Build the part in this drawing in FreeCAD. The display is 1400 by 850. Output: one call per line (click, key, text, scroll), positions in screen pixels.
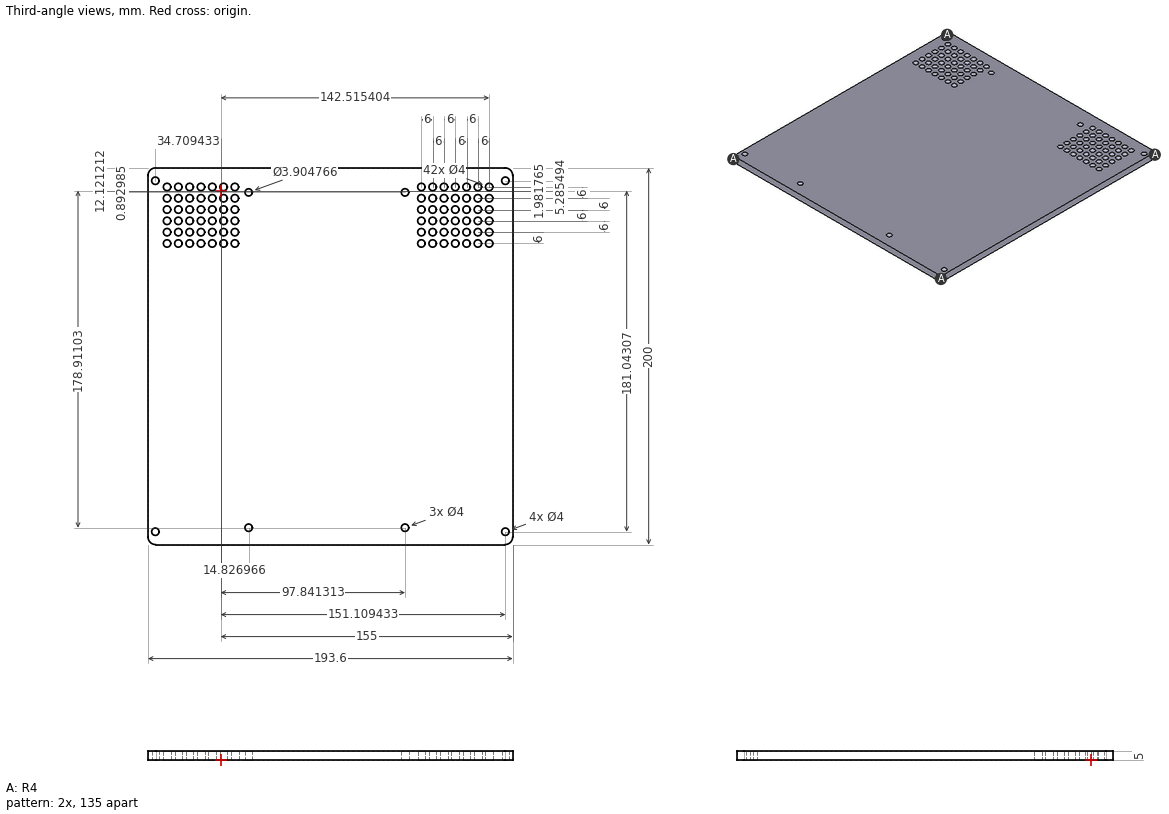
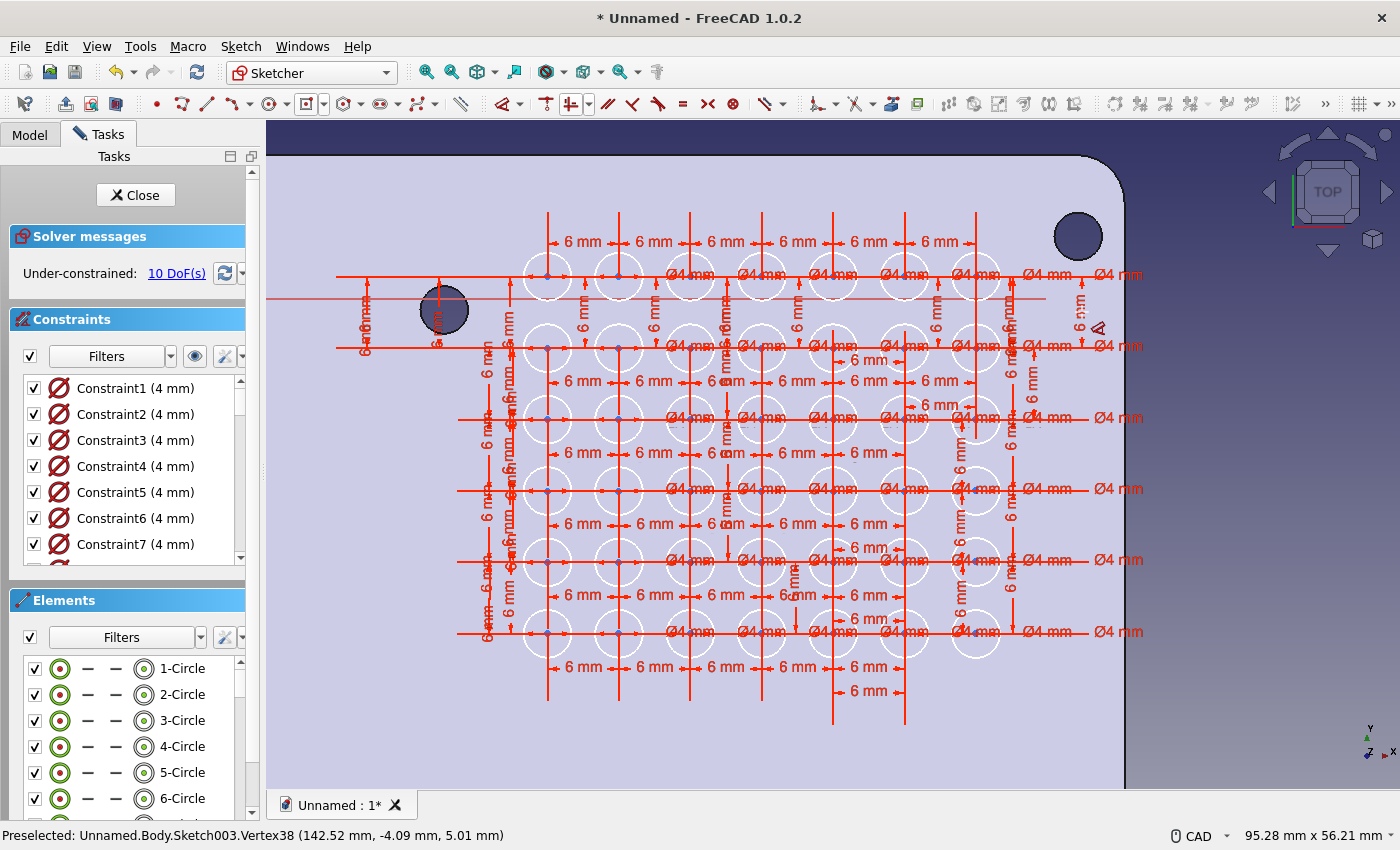
click(905, 420)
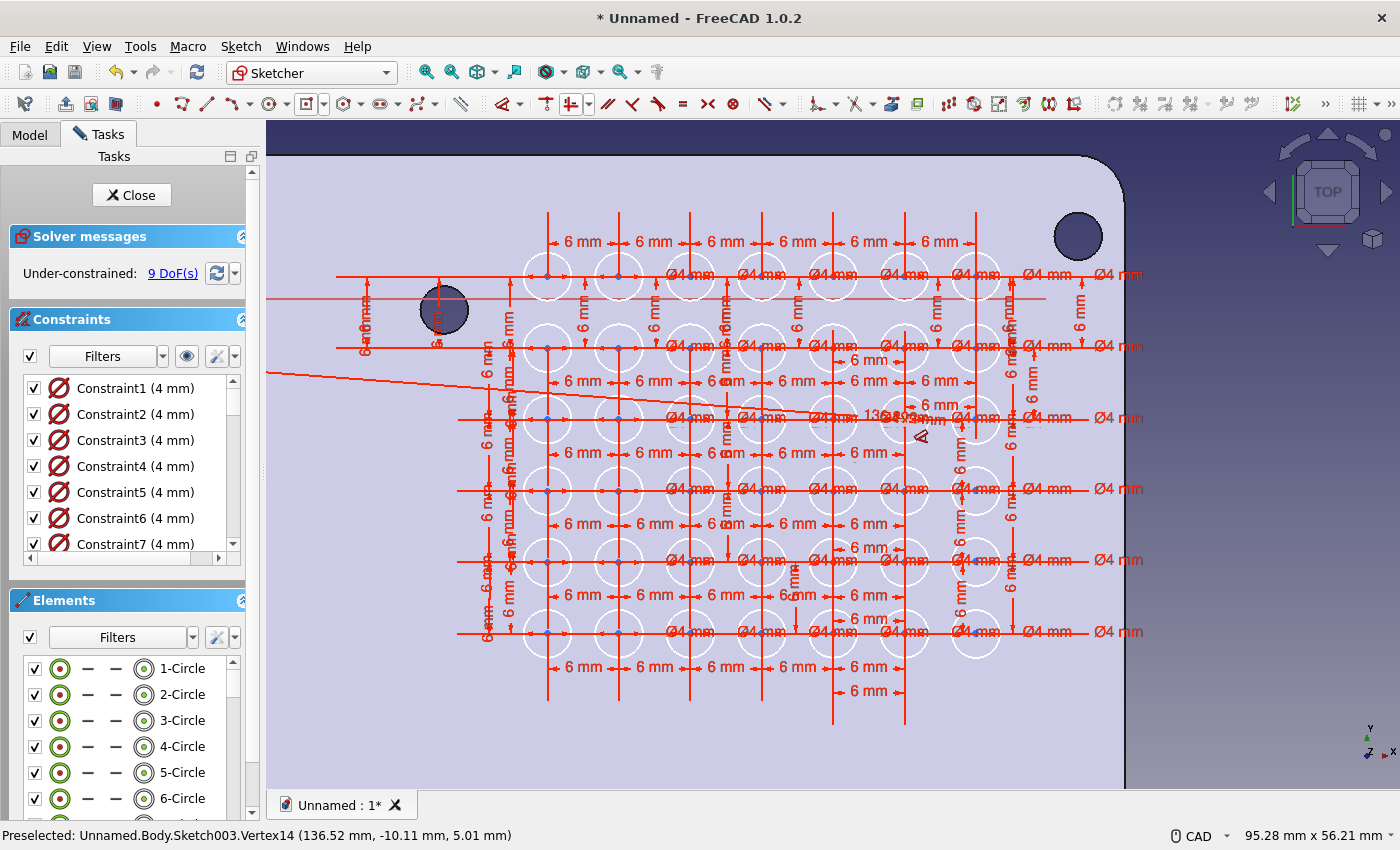
click(976, 420)
click(940, 362)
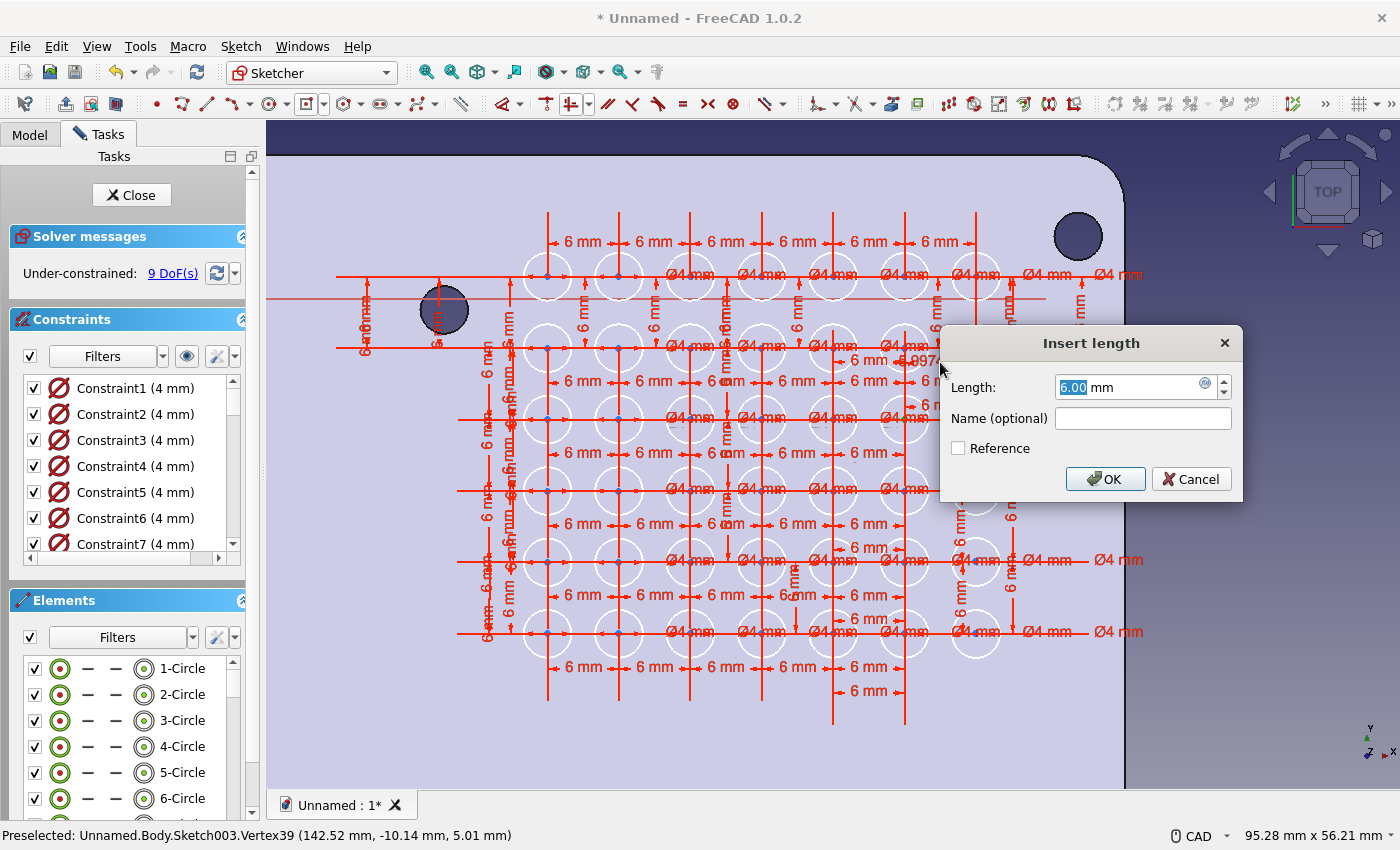
text(6)
key(Return)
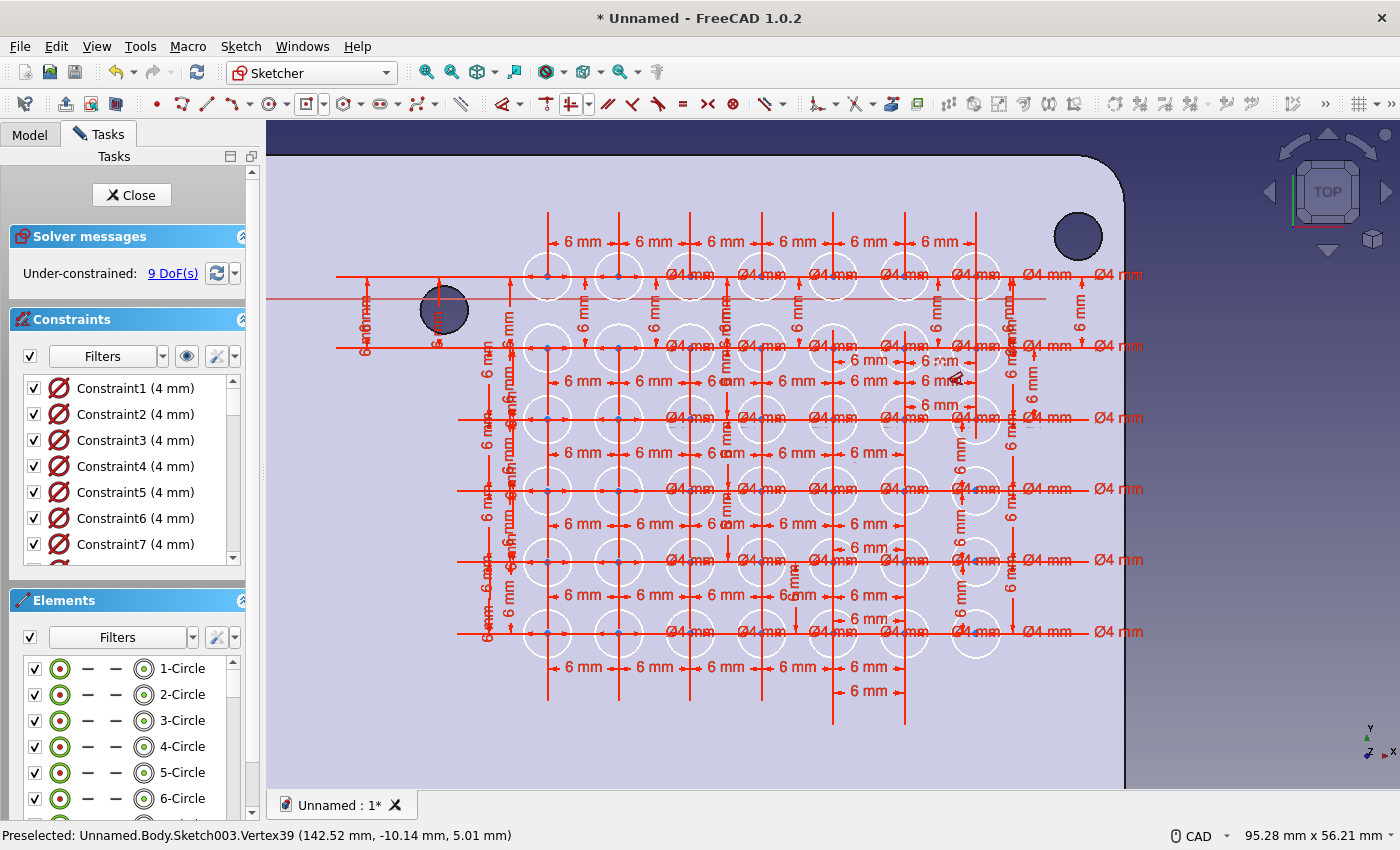
click(976, 348)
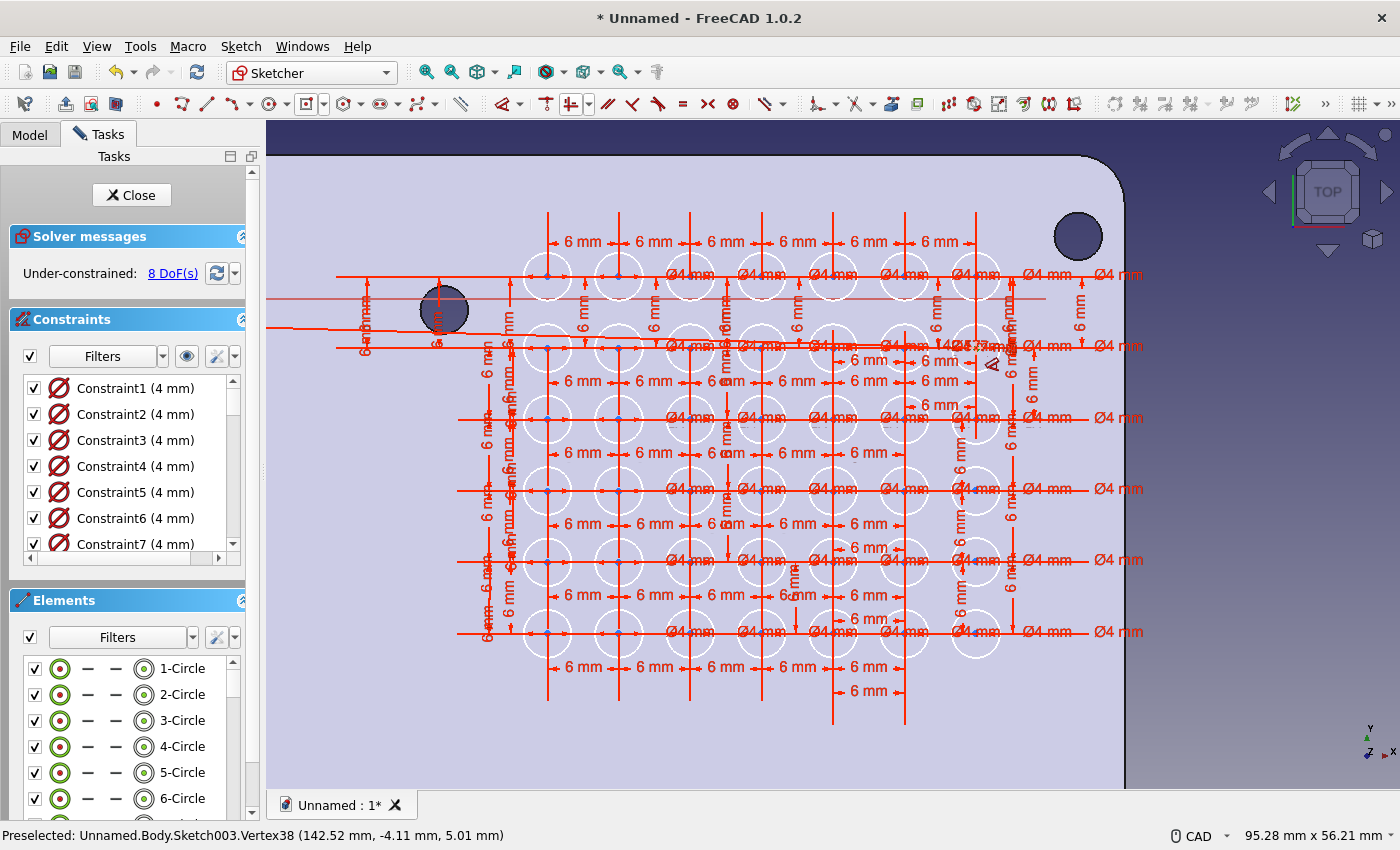
click(976, 420)
click(1034, 409)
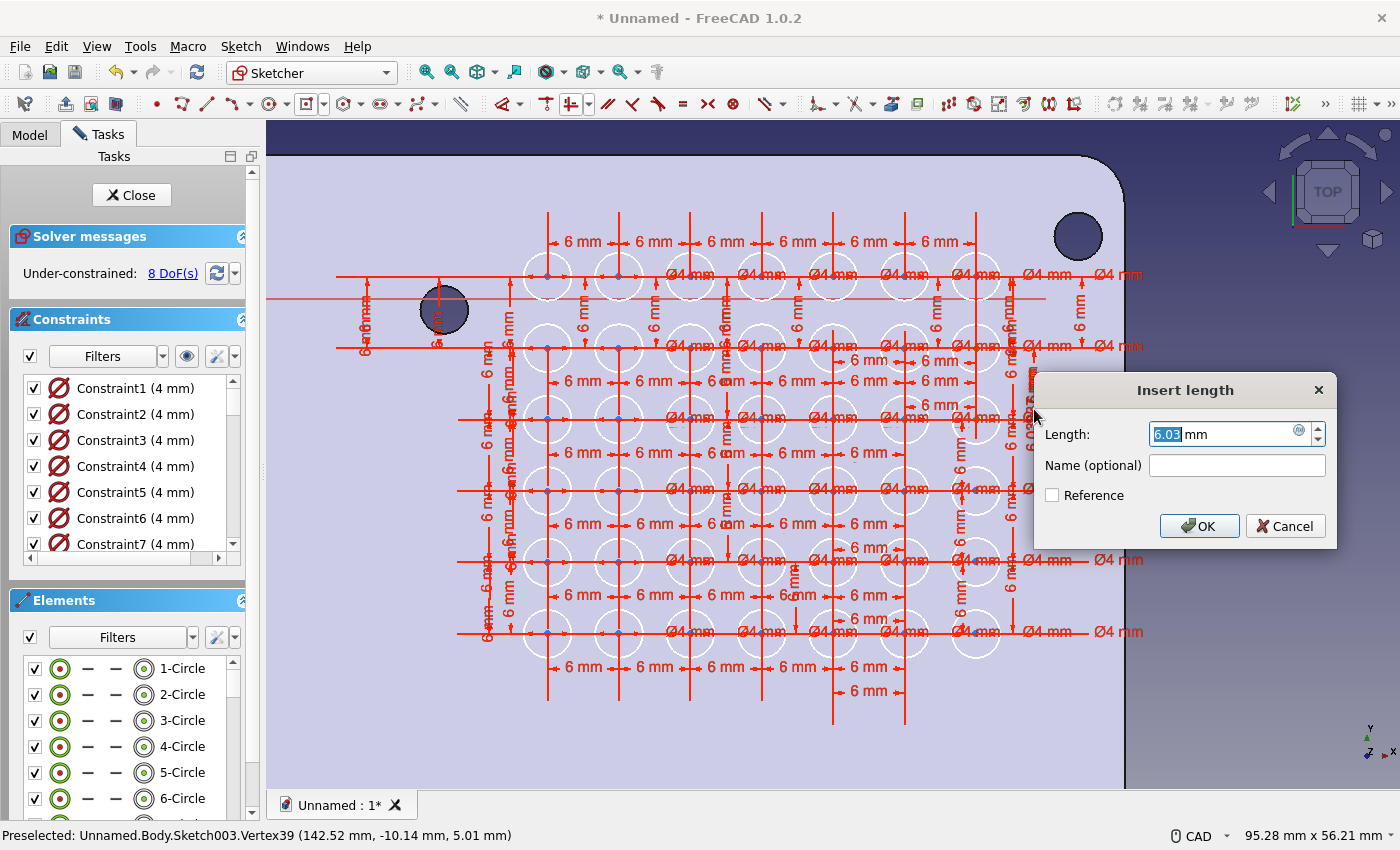
text(6)
key(Return)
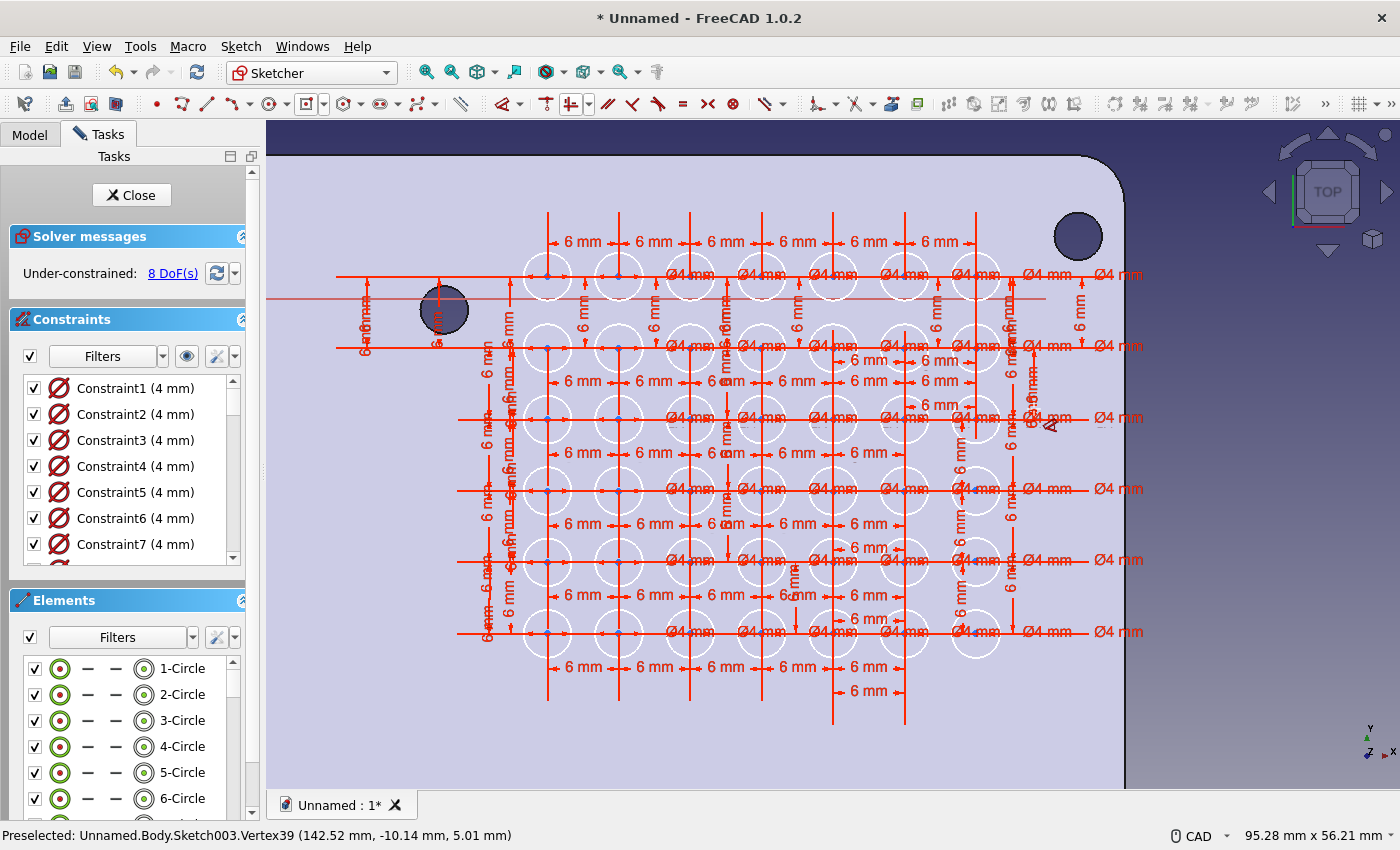
click(905, 491)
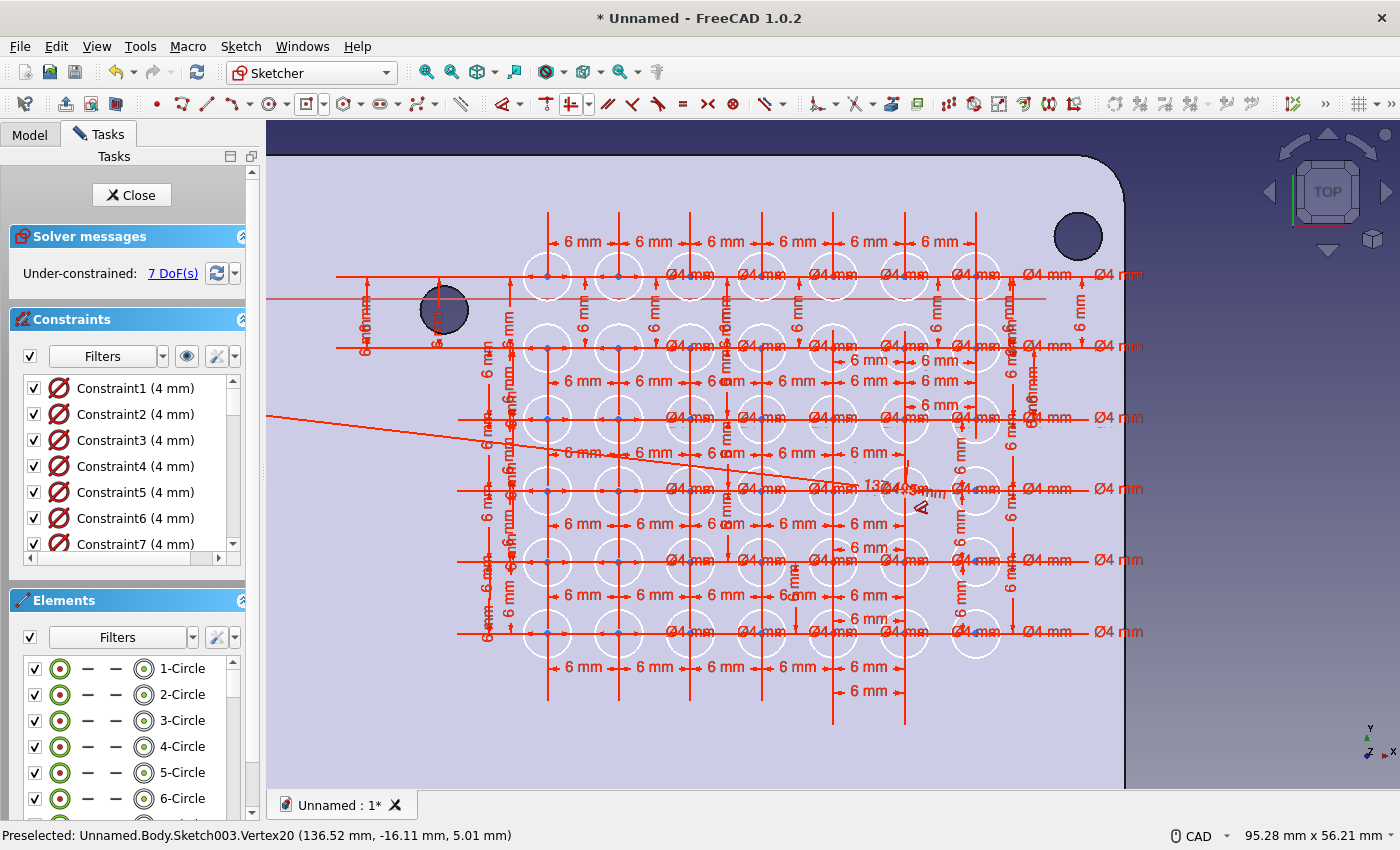
click(976, 491)
click(940, 549)